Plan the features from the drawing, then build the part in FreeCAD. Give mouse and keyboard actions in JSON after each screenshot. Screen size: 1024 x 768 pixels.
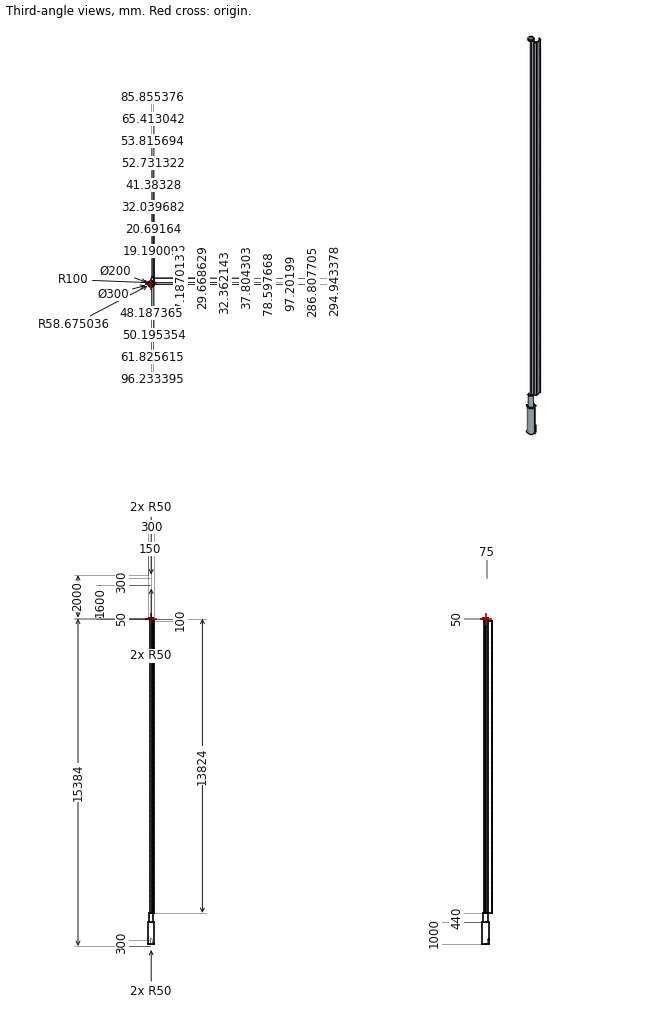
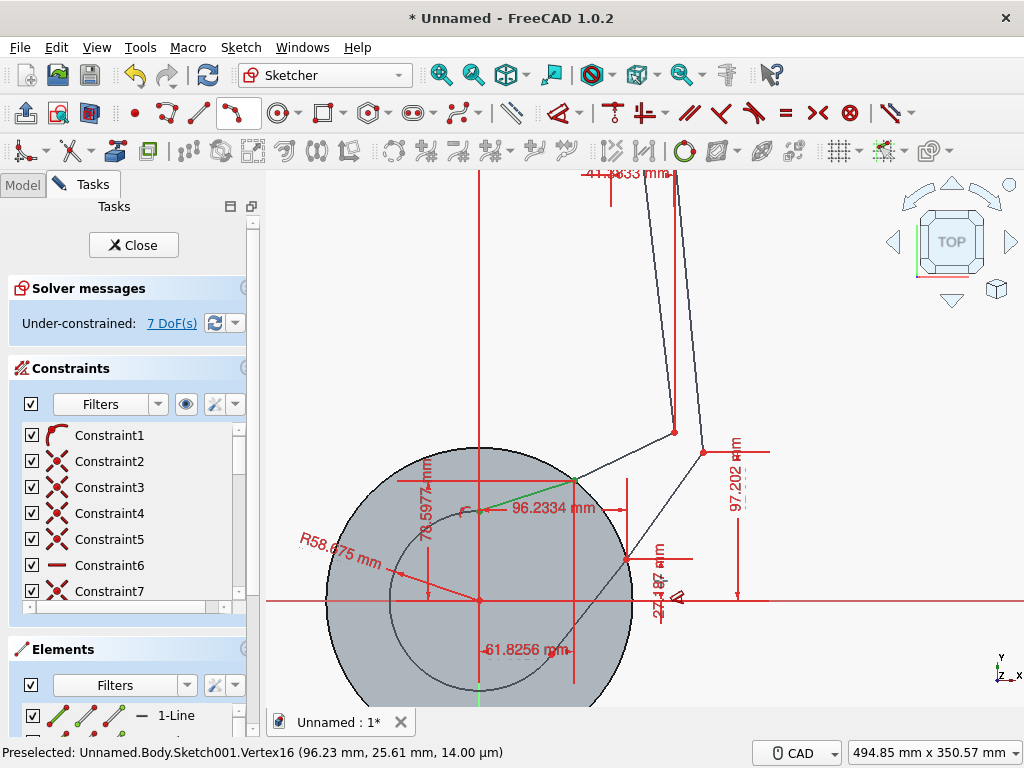
{"action": "left_click", "coordinate": [551, 655]}
{"action": "left_click", "coordinate": [515, 567]}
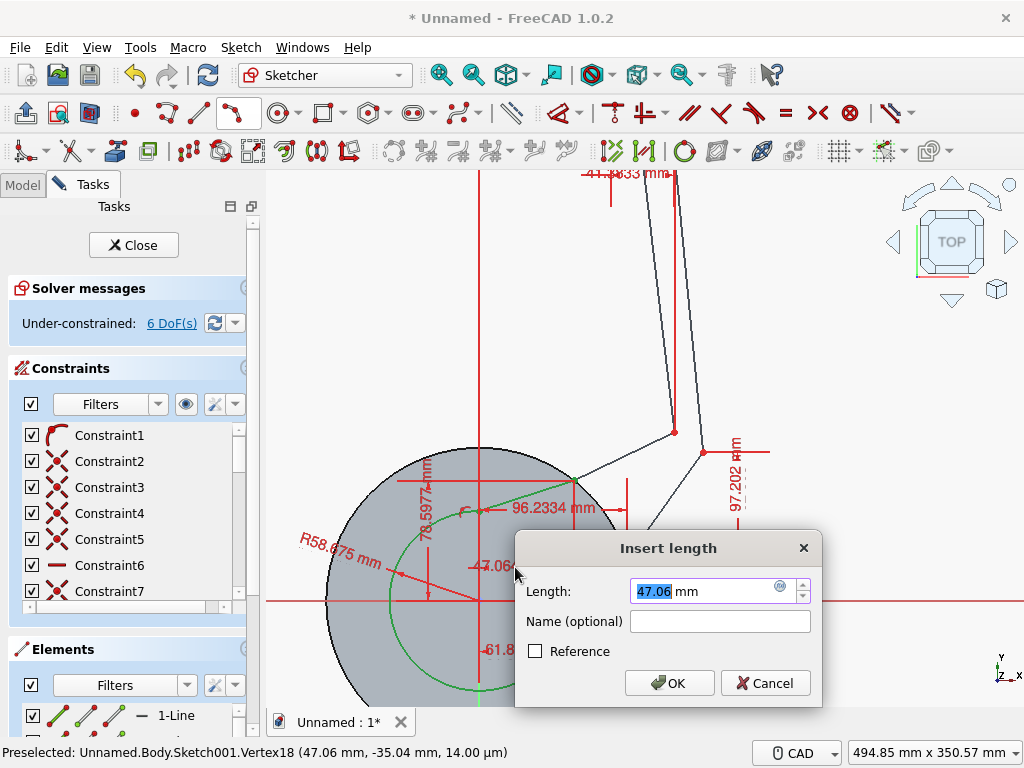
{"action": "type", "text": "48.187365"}
{"action": "key", "text": "Return"}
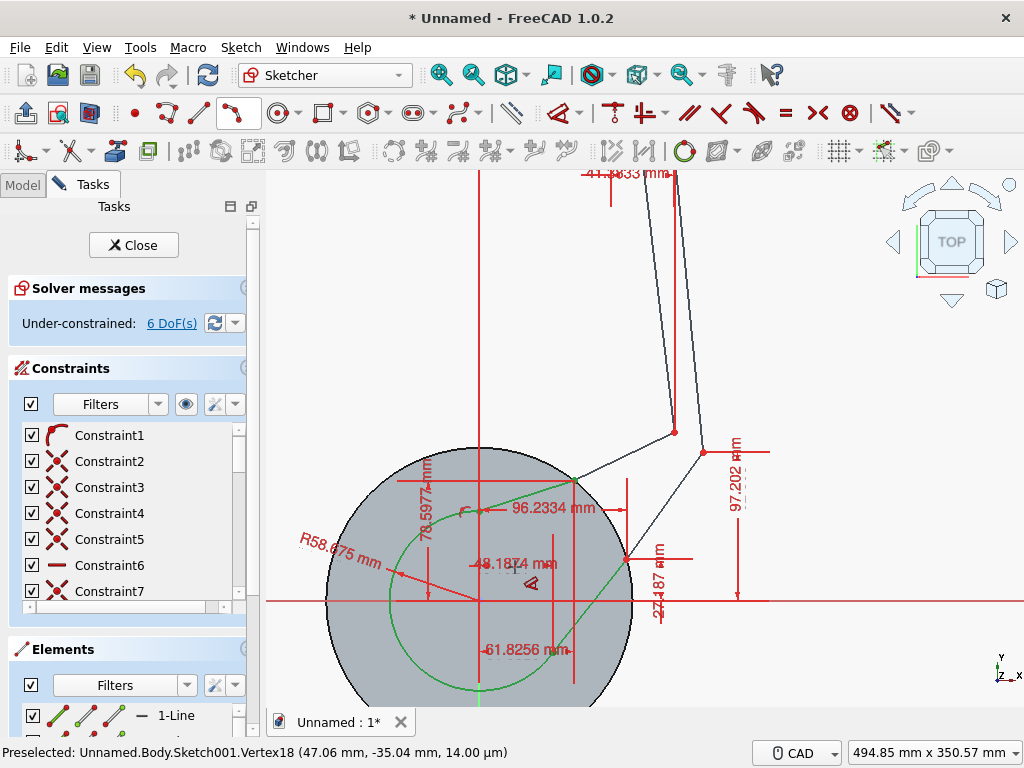
{"action": "left_click", "coordinate": [604, 466]}
{"action": "left_click", "coordinate": [624, 515]}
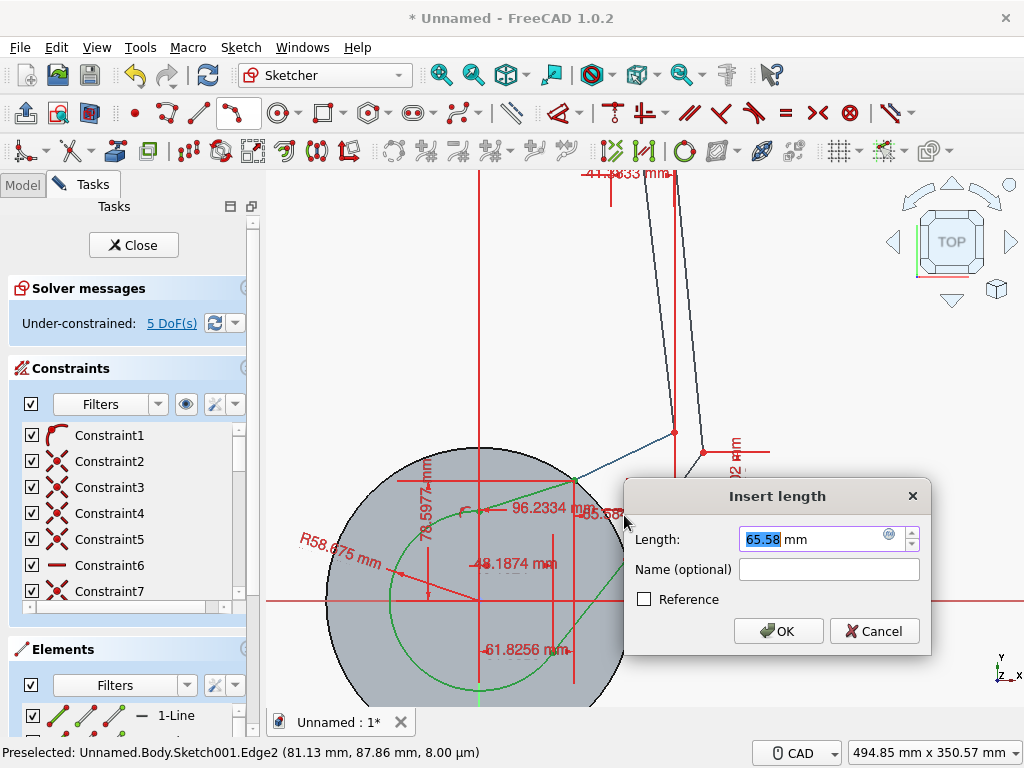
{"action": "type", "text": "65.413042"}
{"action": "key", "text": "Return"}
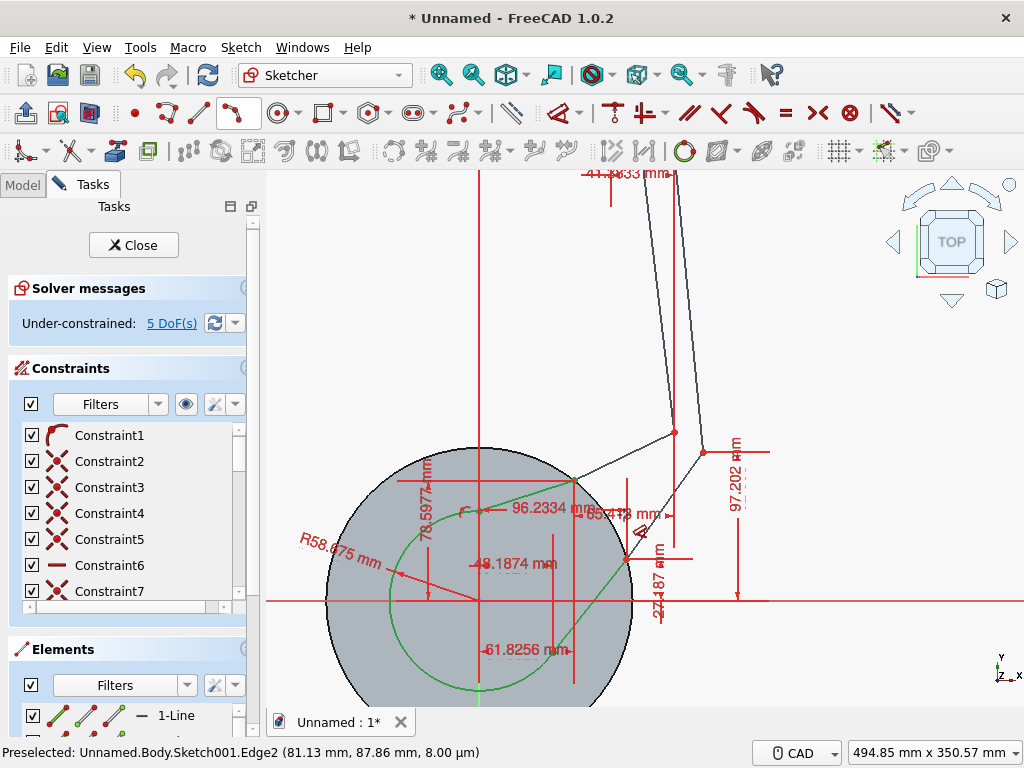
{"action": "left_click", "coordinate": [604, 466]}
{"action": "left_click", "coordinate": [540, 456]}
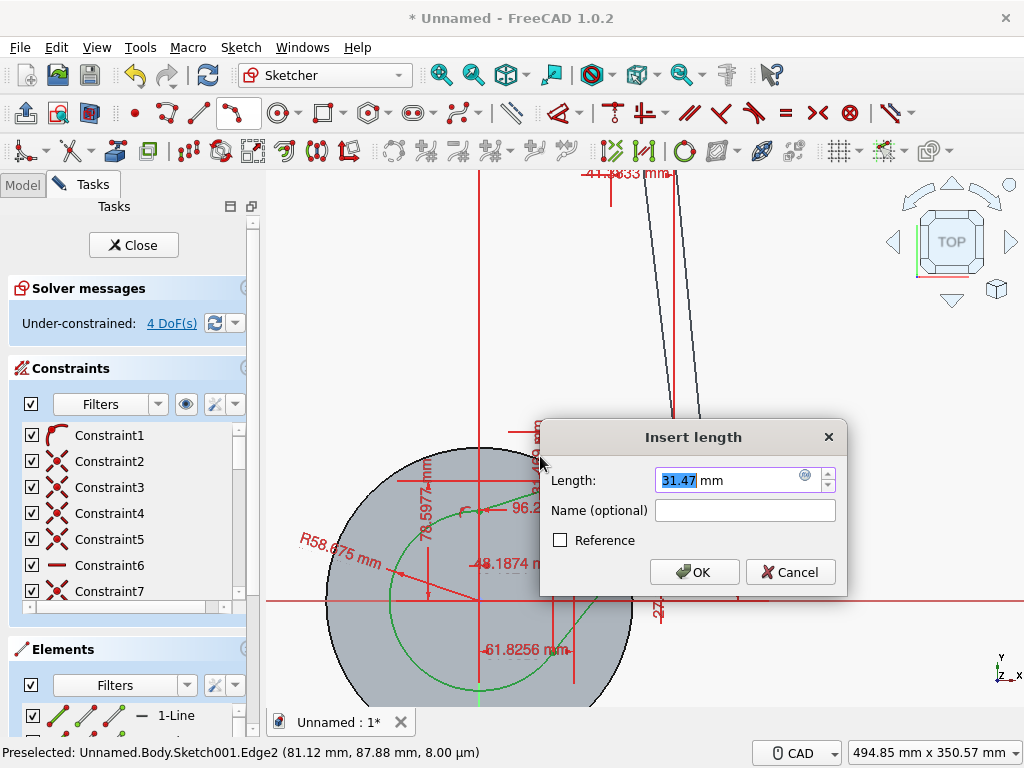
{"action": "type", "text": "32.362143"}
{"action": "key", "text": "Return"}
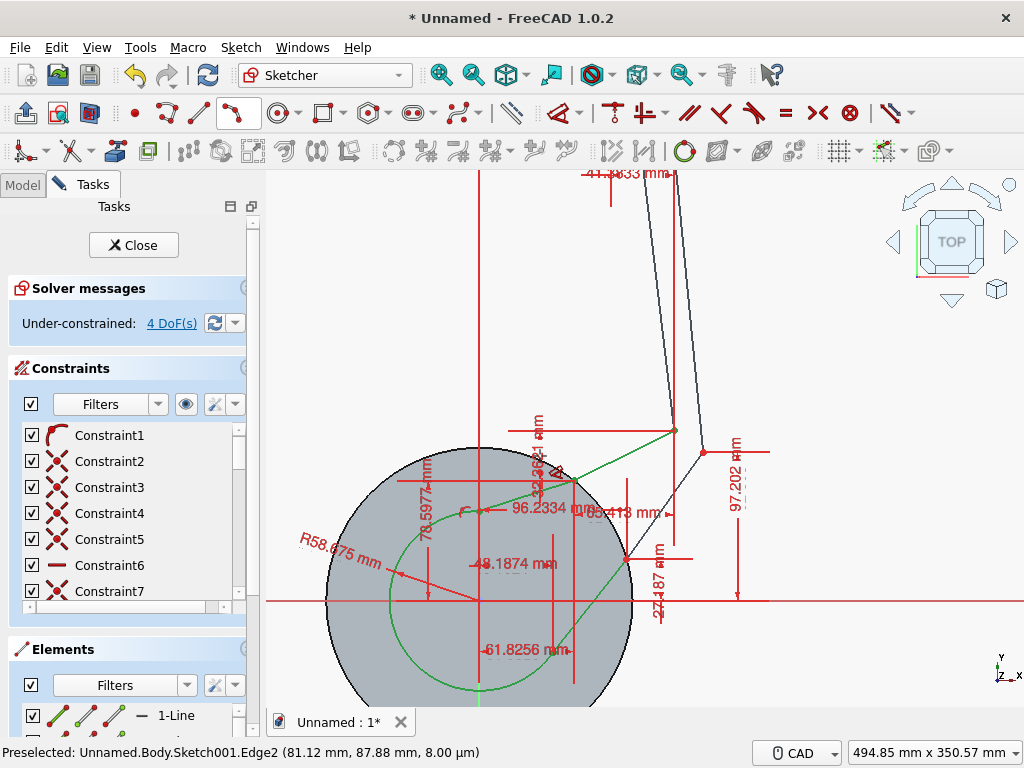
{"action": "scroll", "coordinate": [627, 562], "scroll_direction": "down", "scroll_amount": 2}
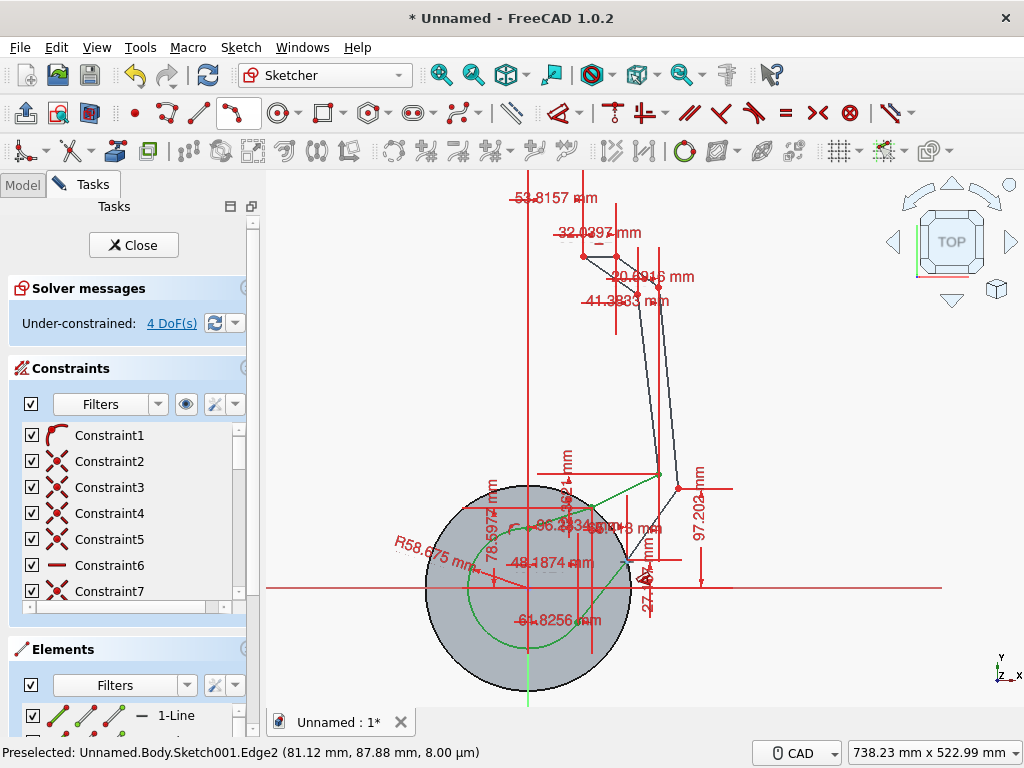
{"action": "left_click", "coordinate": [621, 283]}
{"action": "left_click", "coordinate": [549, 276]}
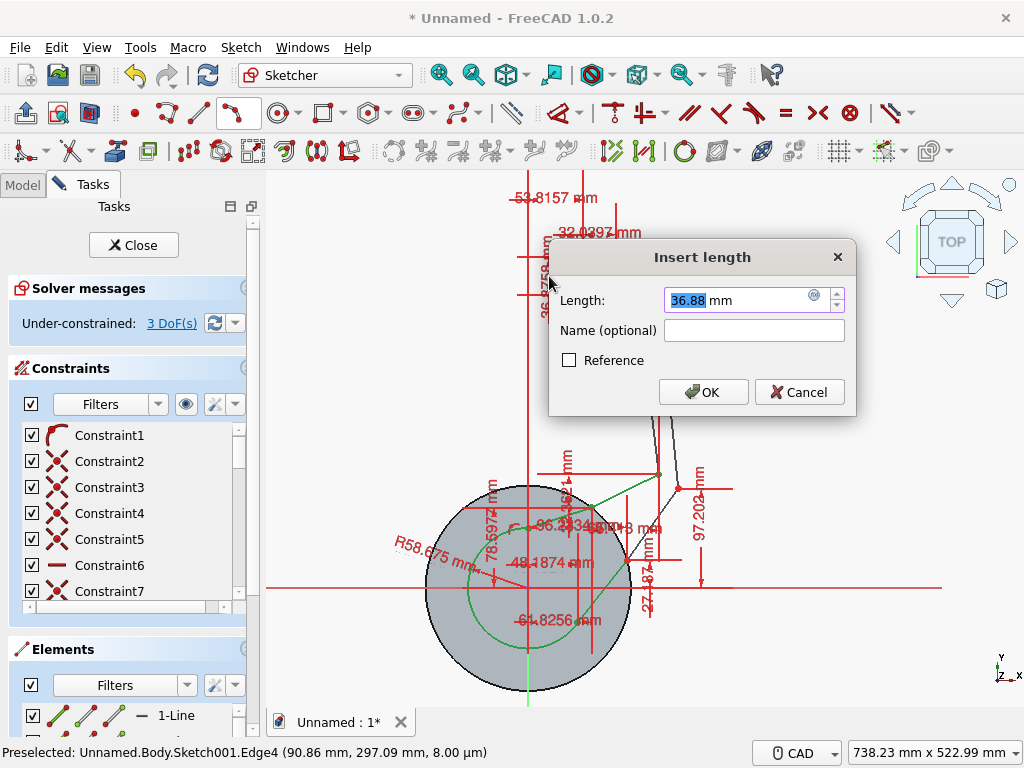
{"action": "type", "text": "37.804303"}
{"action": "key", "text": "Return"}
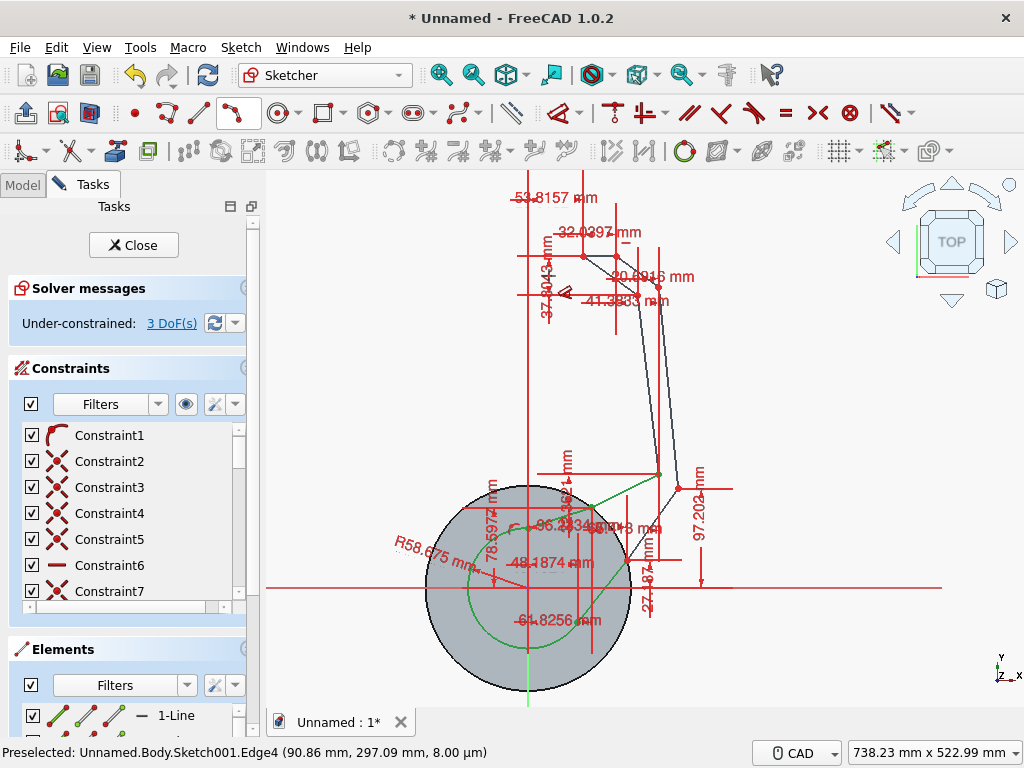
{"action": "scroll", "coordinate": [629, 266], "scroll_direction": "up", "scroll_amount": 2}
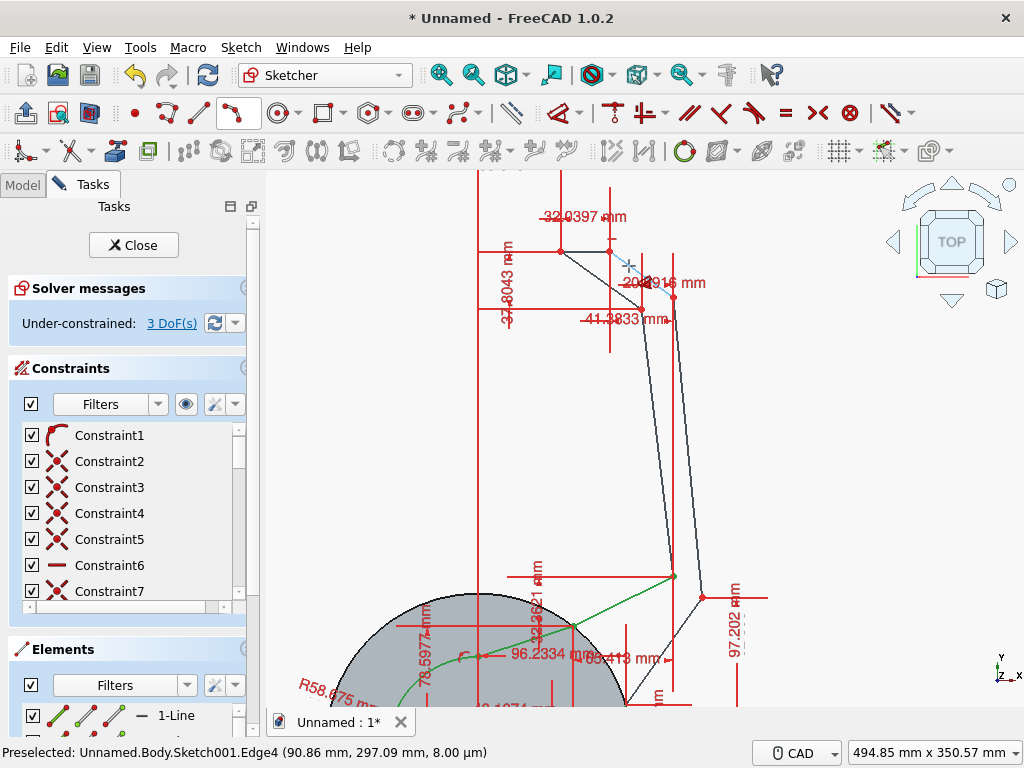
{"action": "left_click", "coordinate": [629, 265]}
{"action": "left_click", "coordinate": [707, 264]}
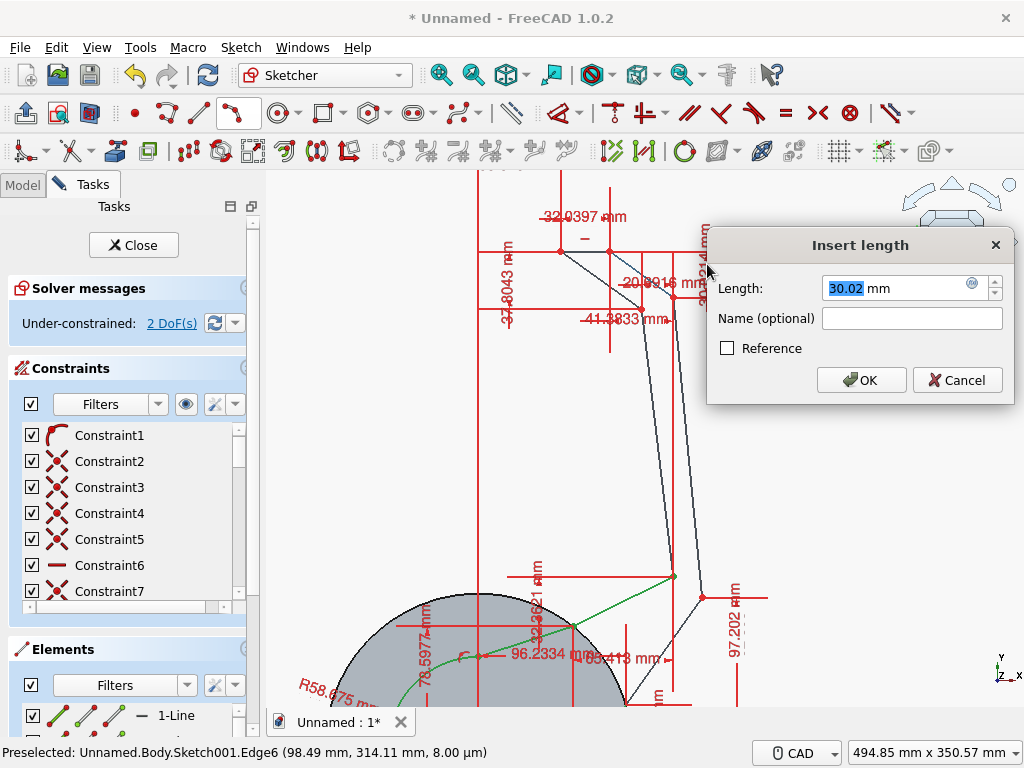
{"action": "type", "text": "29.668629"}
{"action": "key", "text": "Return"}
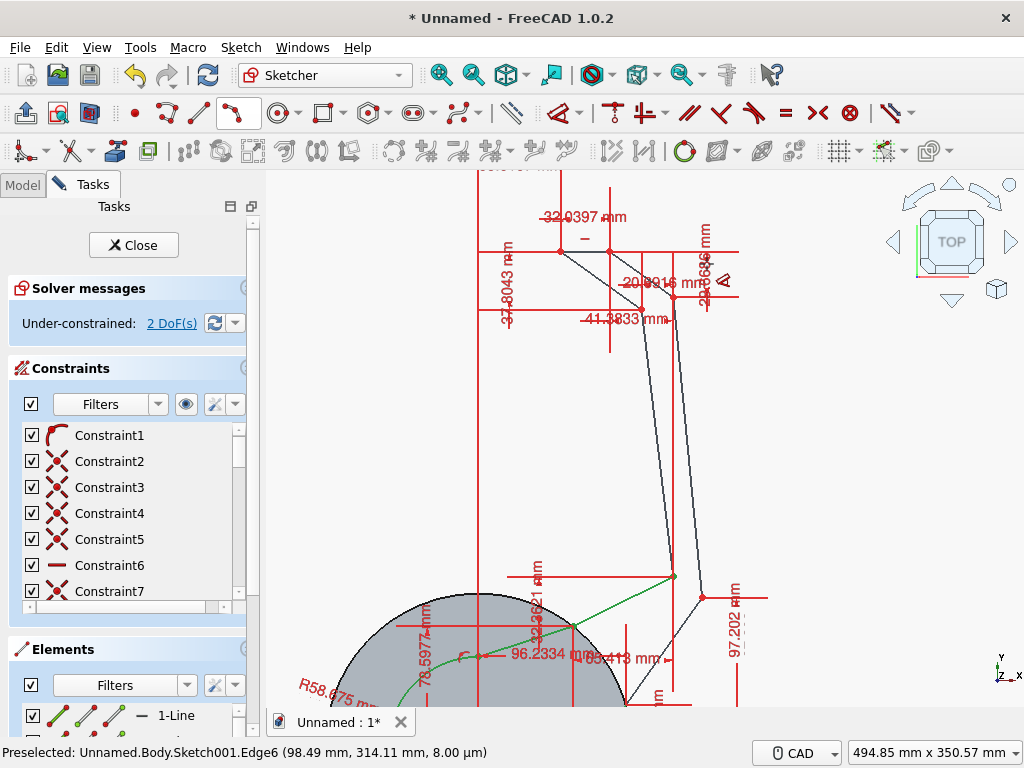
{"action": "scroll", "coordinate": [682, 388], "scroll_direction": "up", "scroll_amount": 2}